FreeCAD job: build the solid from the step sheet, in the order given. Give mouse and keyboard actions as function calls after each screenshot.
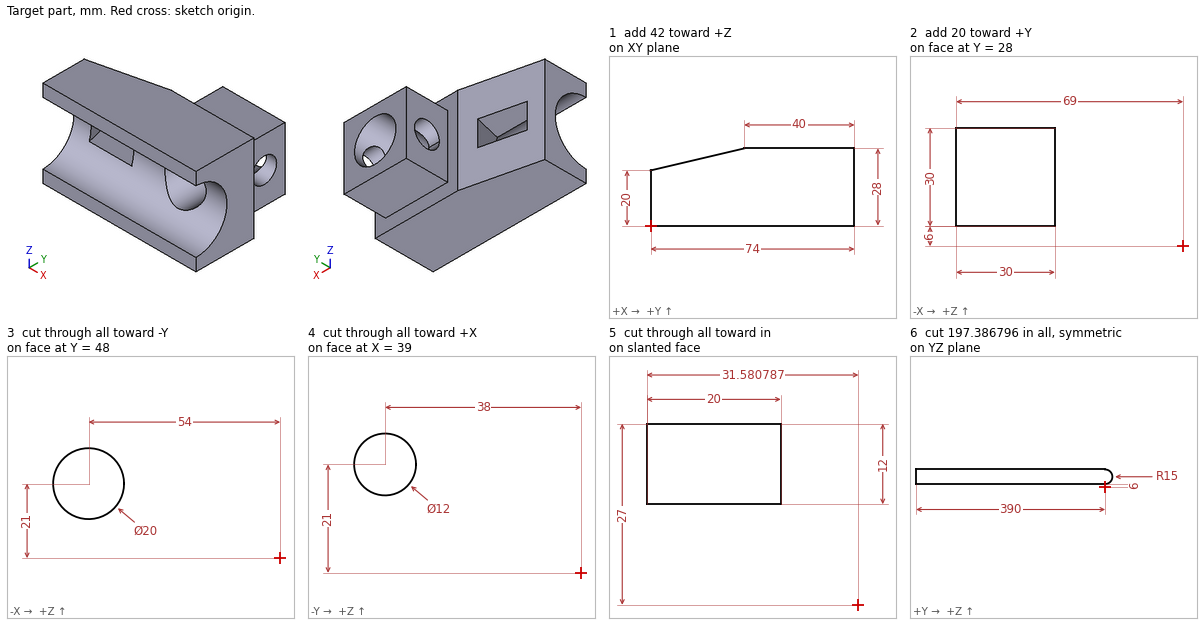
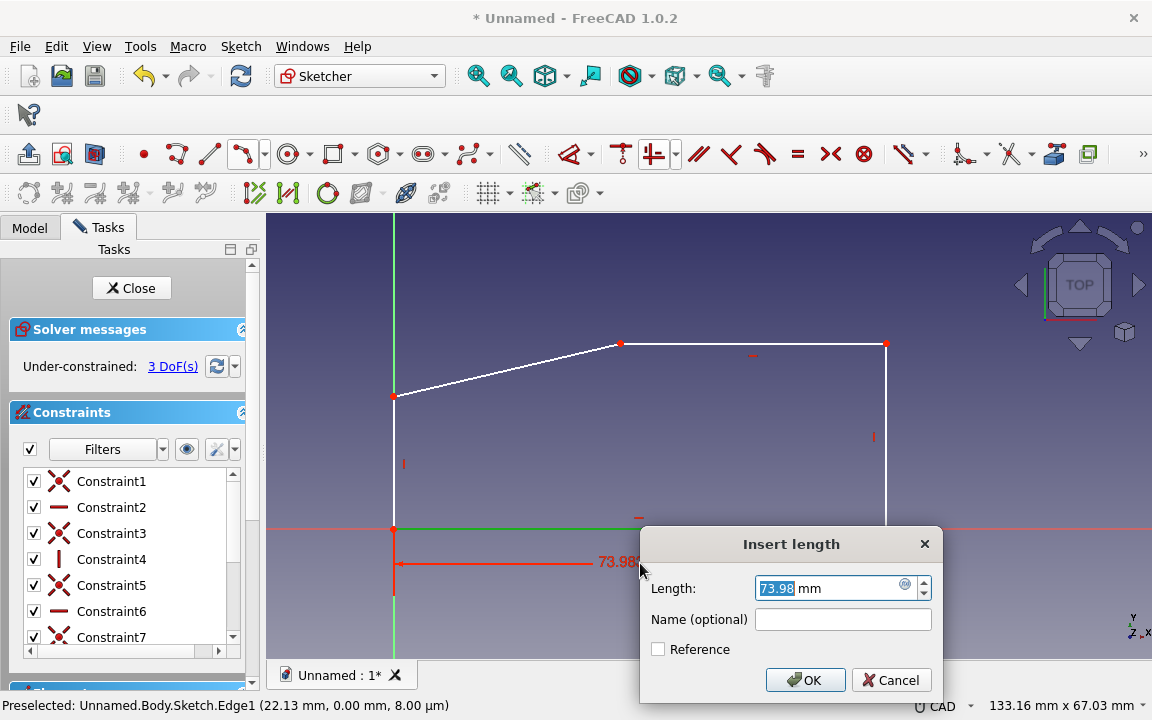
text(74)
key(Return)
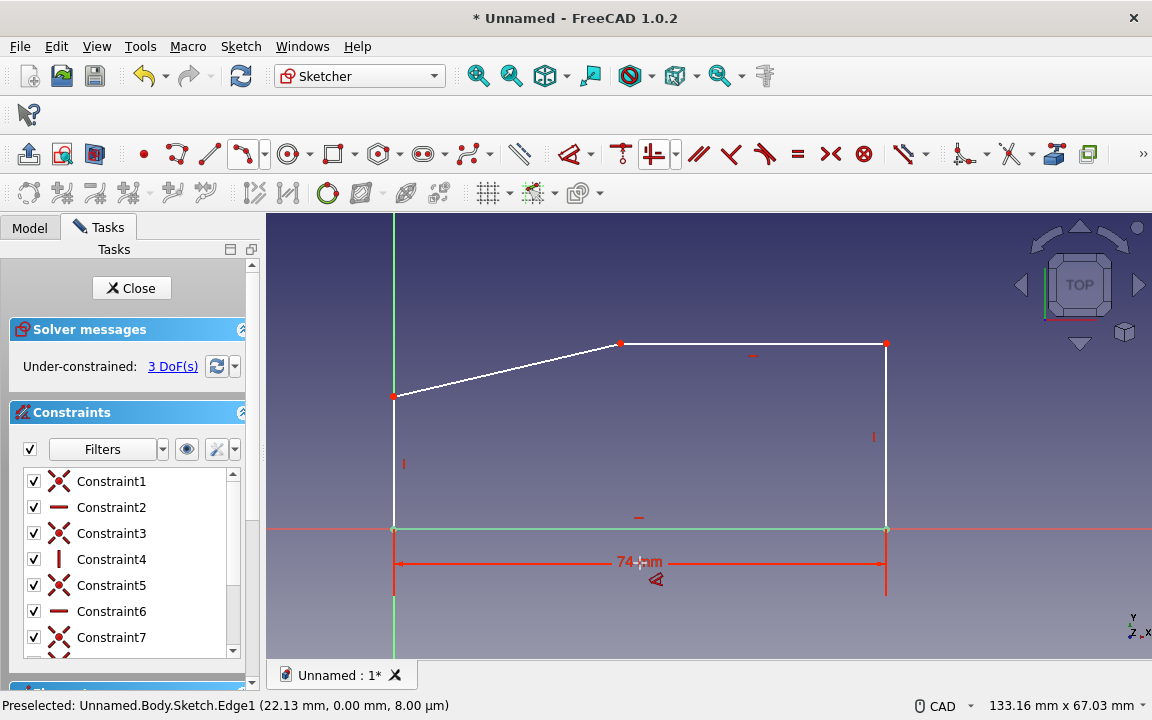
click(886, 474)
click(920, 437)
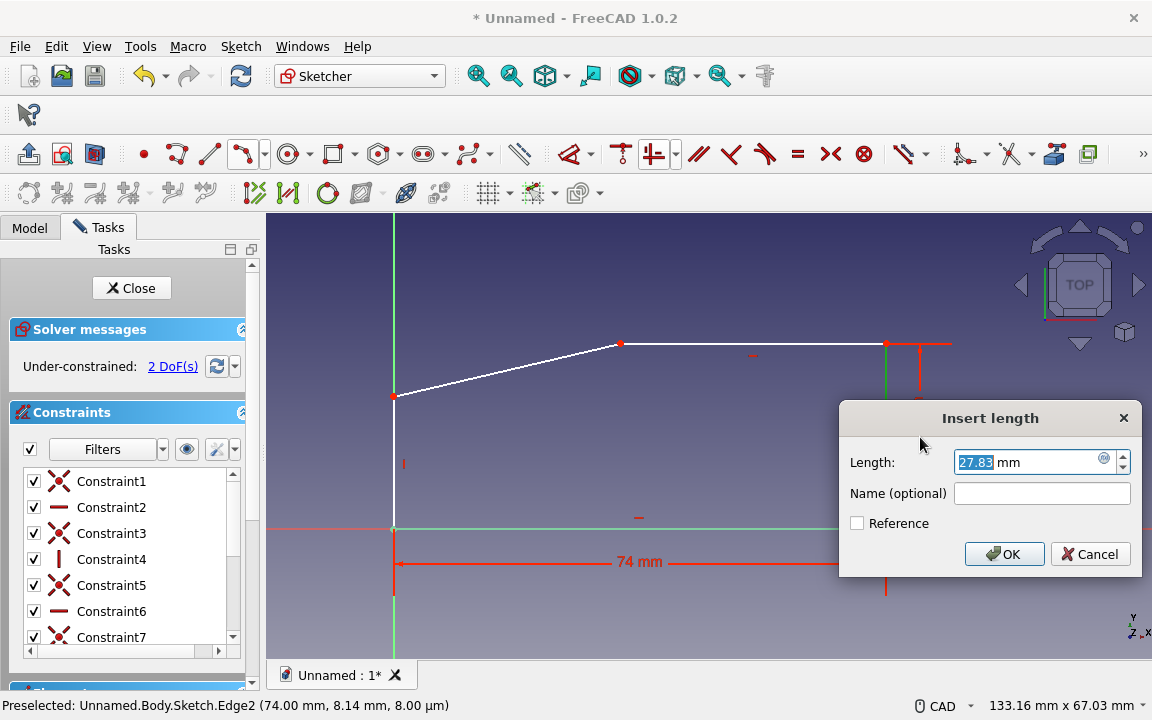
text(28)
key(Return)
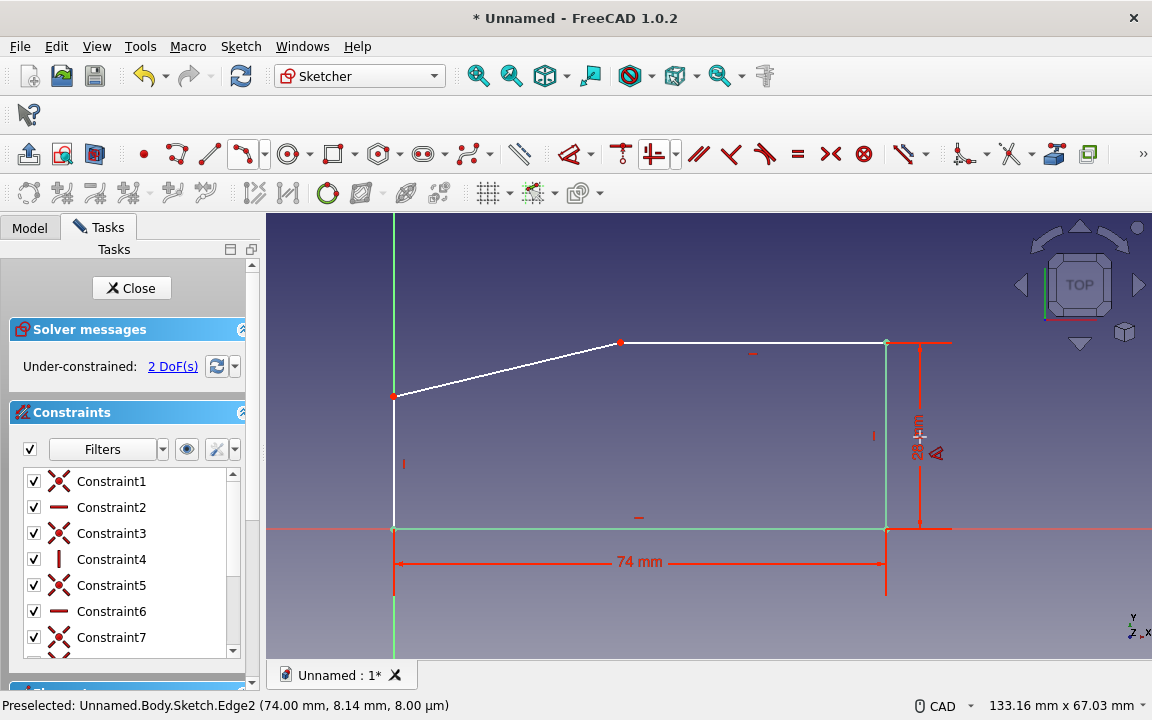
click(806, 343)
click(753, 309)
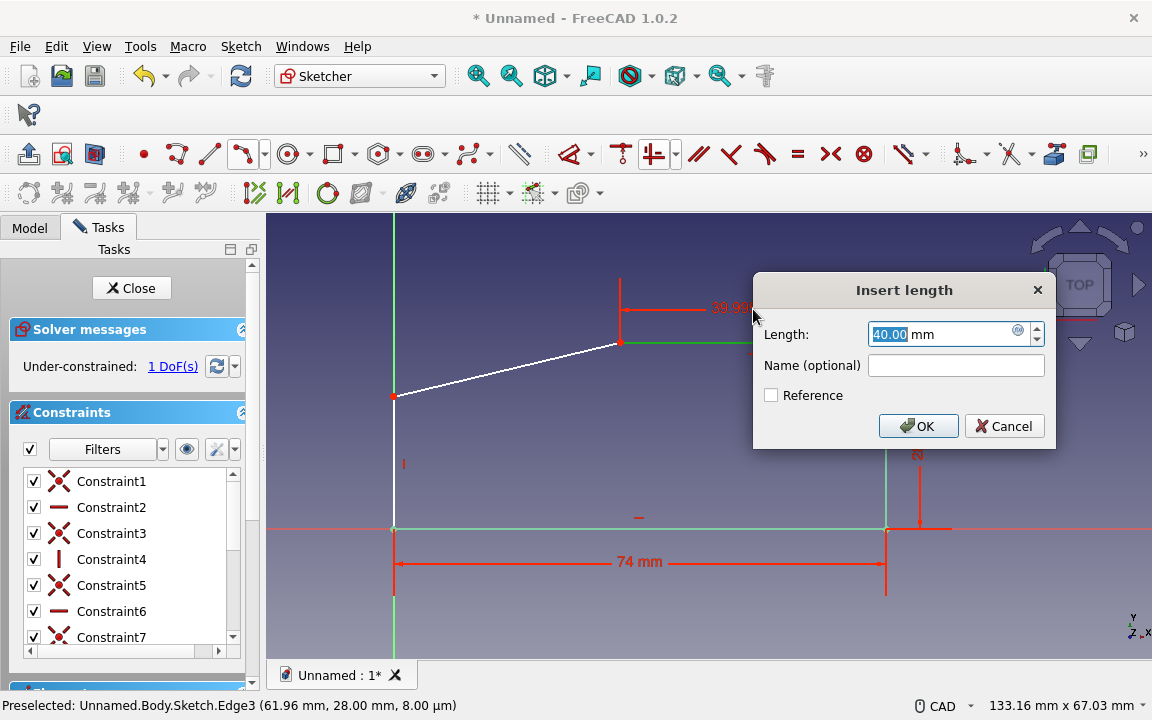
text(40)
key(Return)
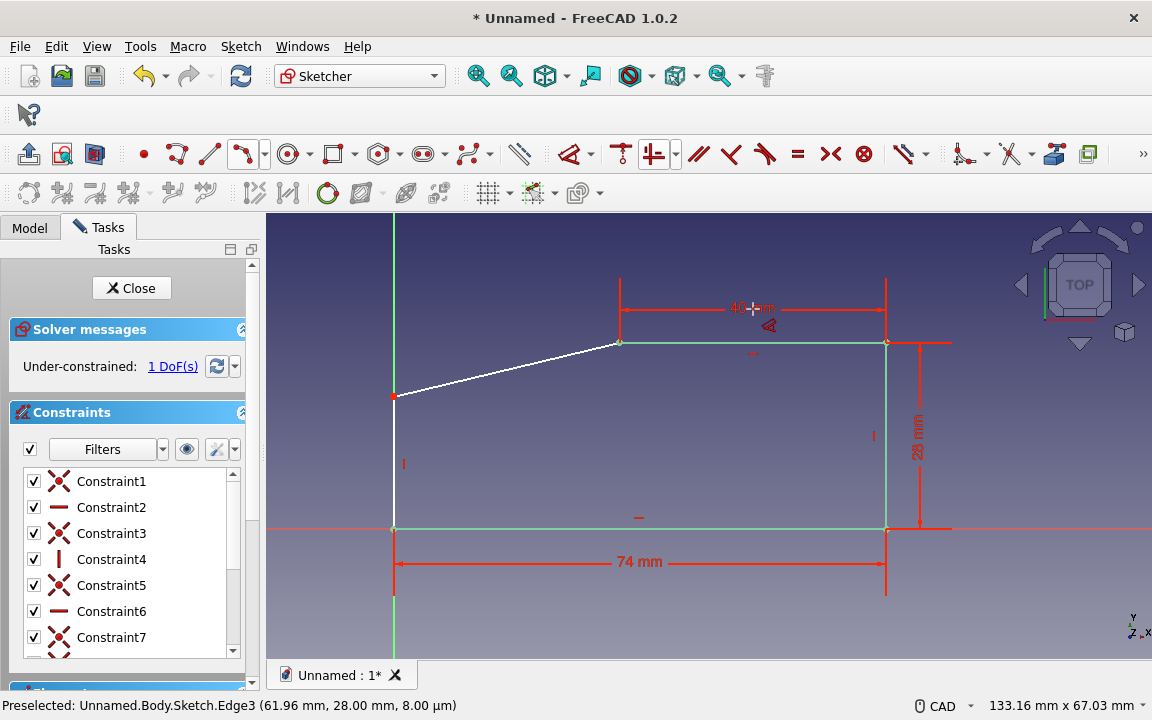
click(394, 437)
click(360, 463)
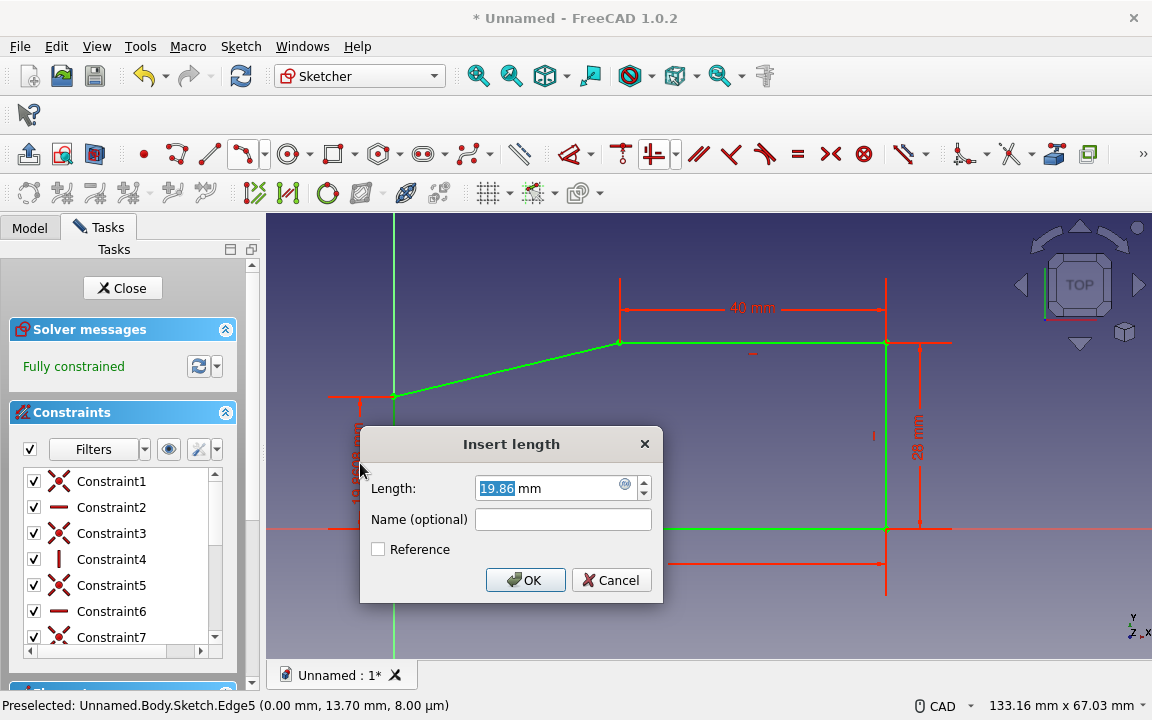
text(20)
key(Return)
key(Escape)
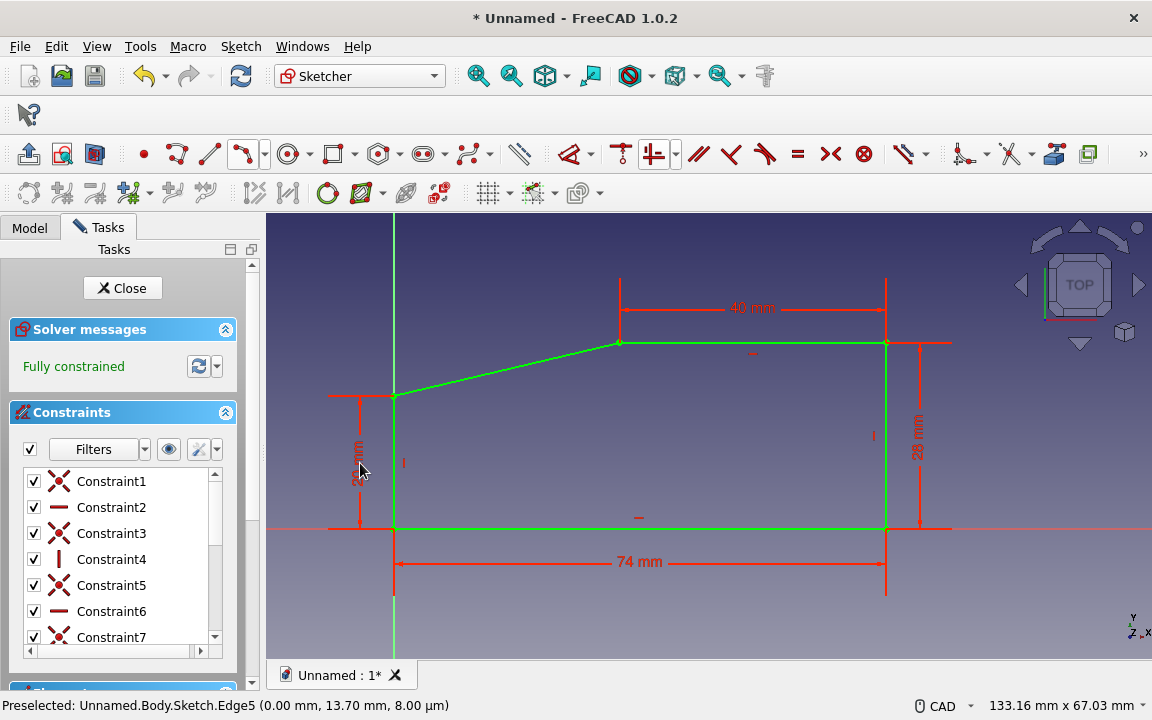
click(123, 288)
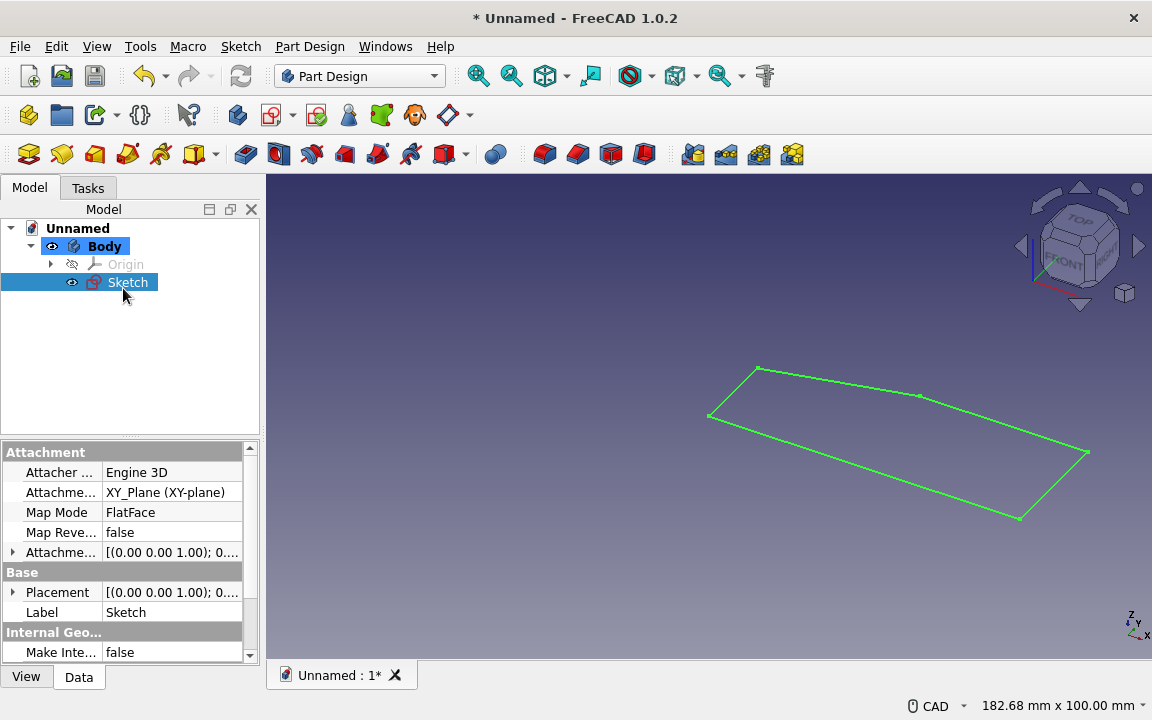
click(29, 154)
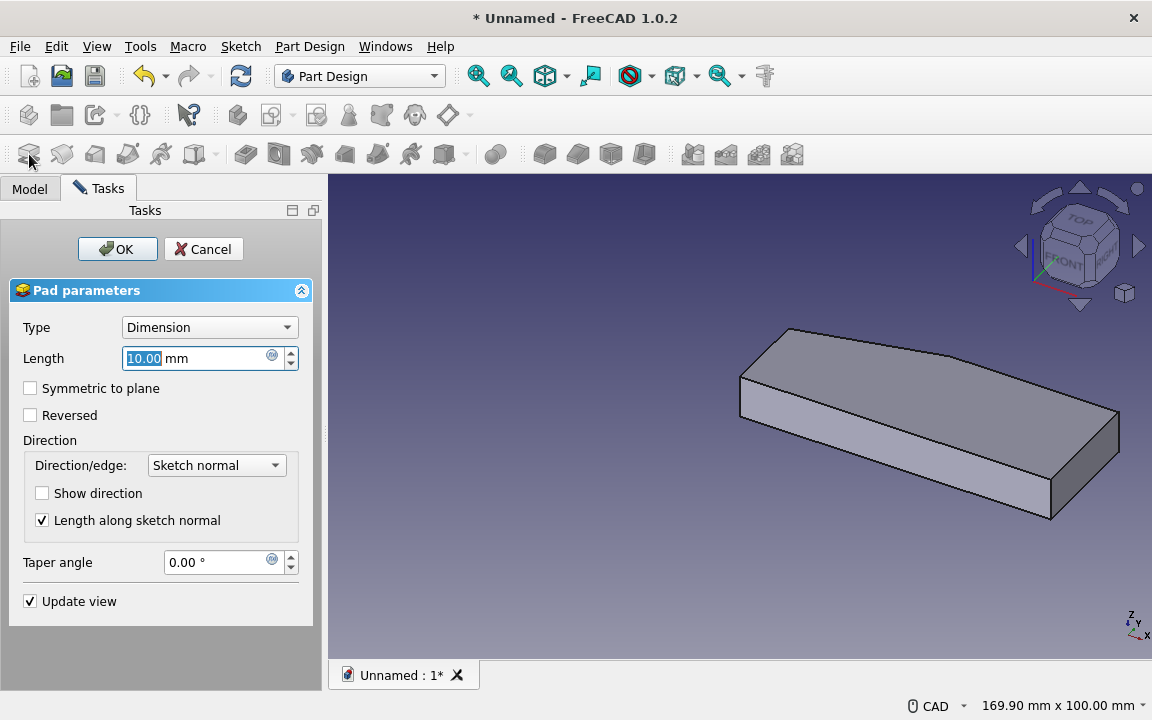
text(42)
key(Tab)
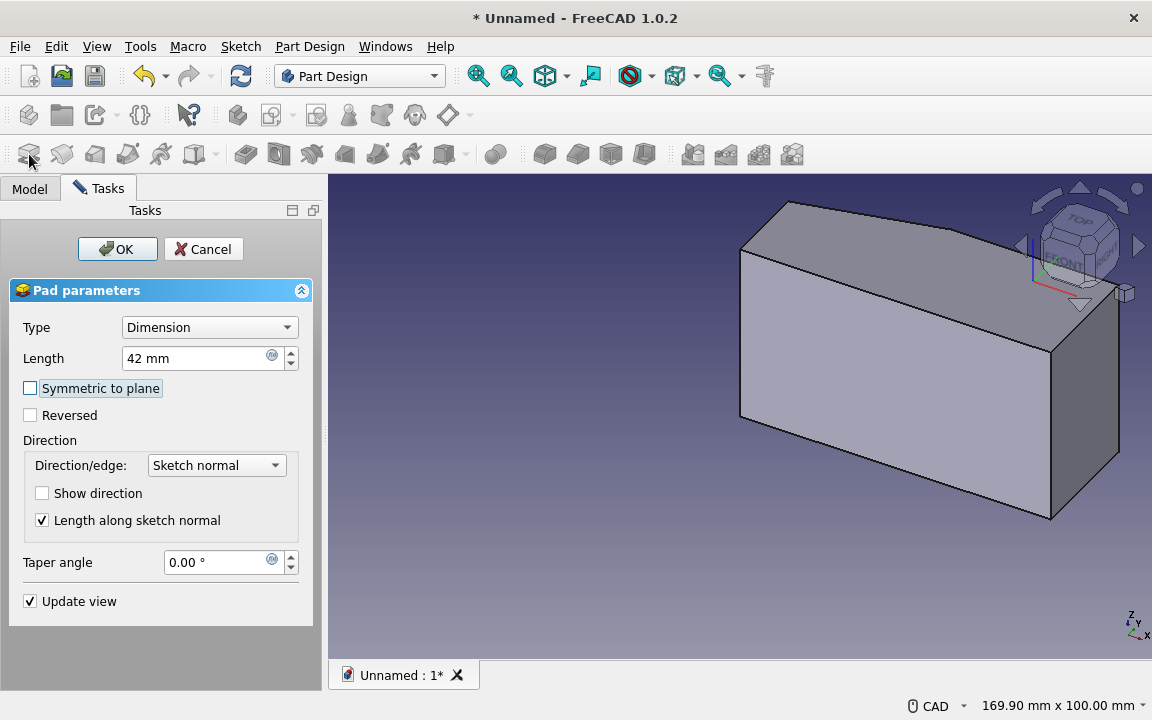
click(118, 249)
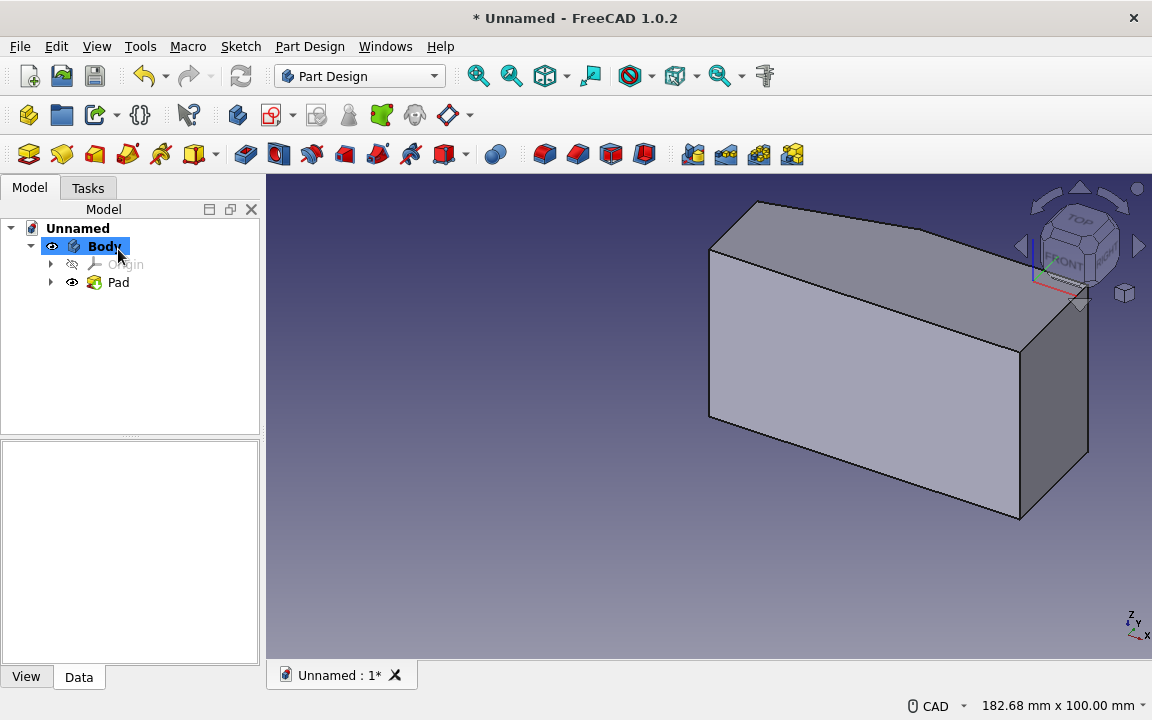
key(4)